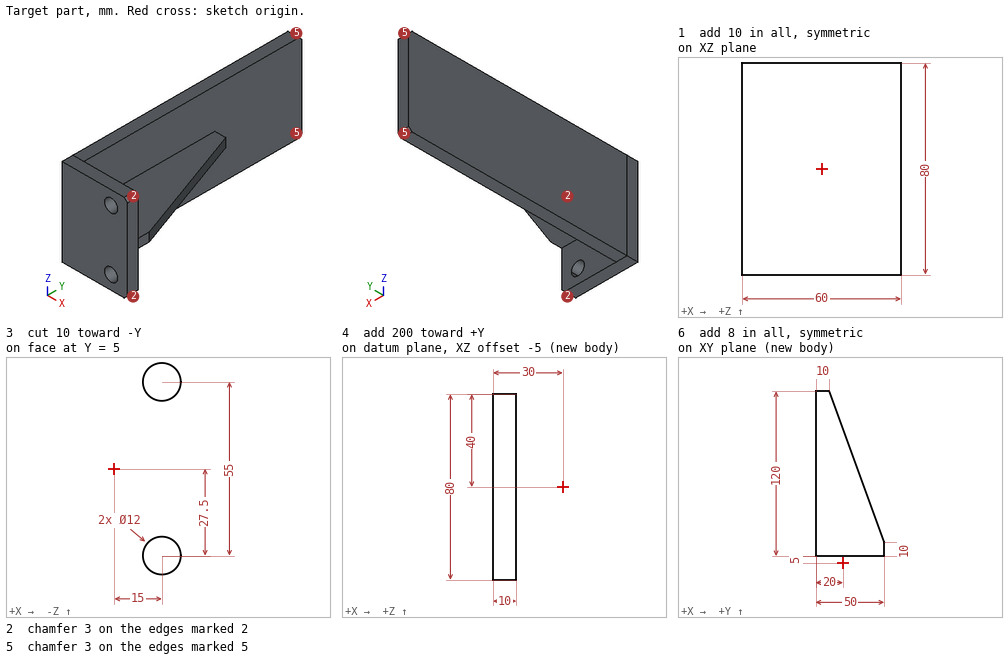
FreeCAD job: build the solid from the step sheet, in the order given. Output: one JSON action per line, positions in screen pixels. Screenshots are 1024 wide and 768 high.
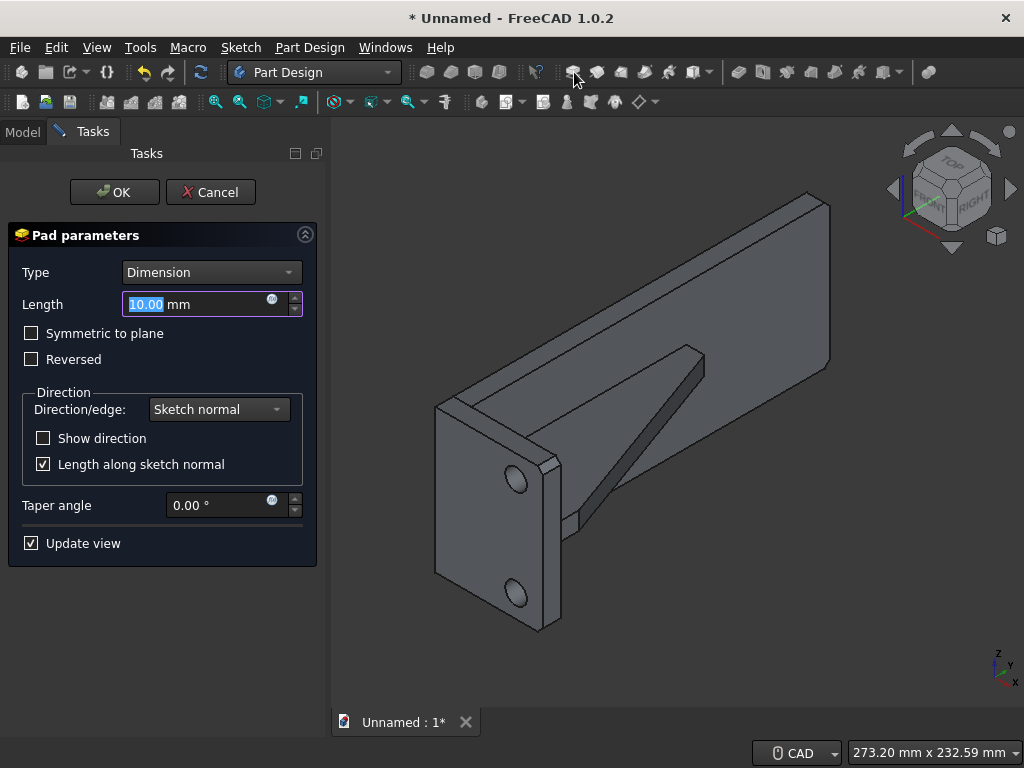
{"action": "type", "text": "8"}
{"action": "key", "text": "Tab"}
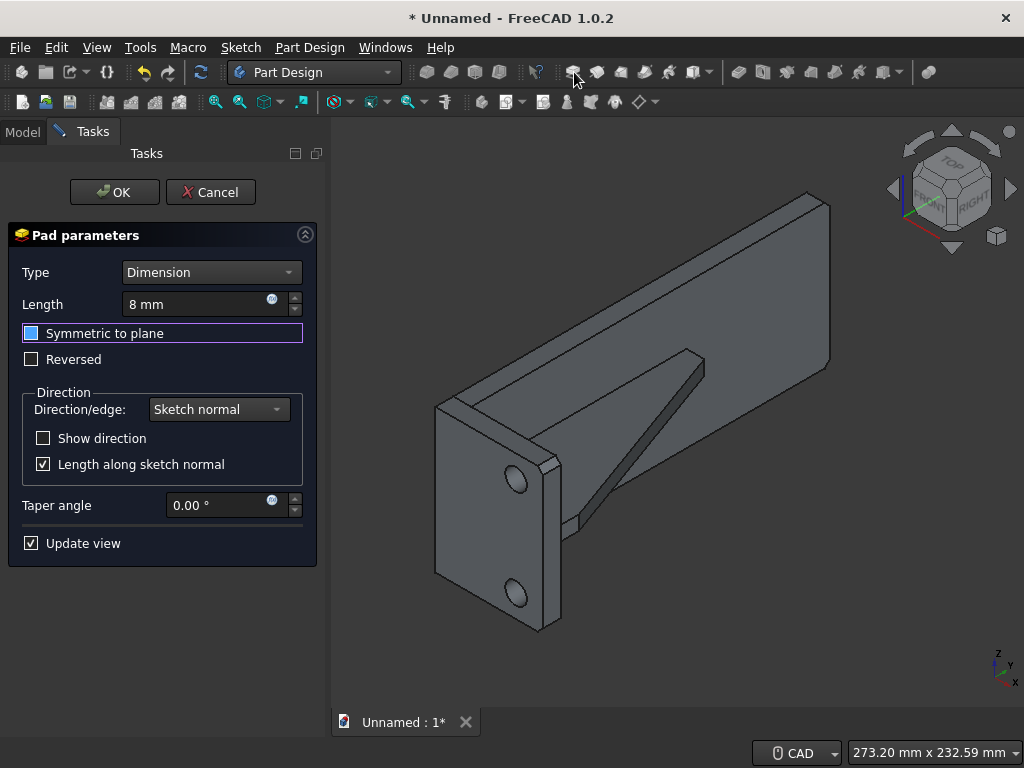
{"action": "left_click", "coordinate": [30, 333]}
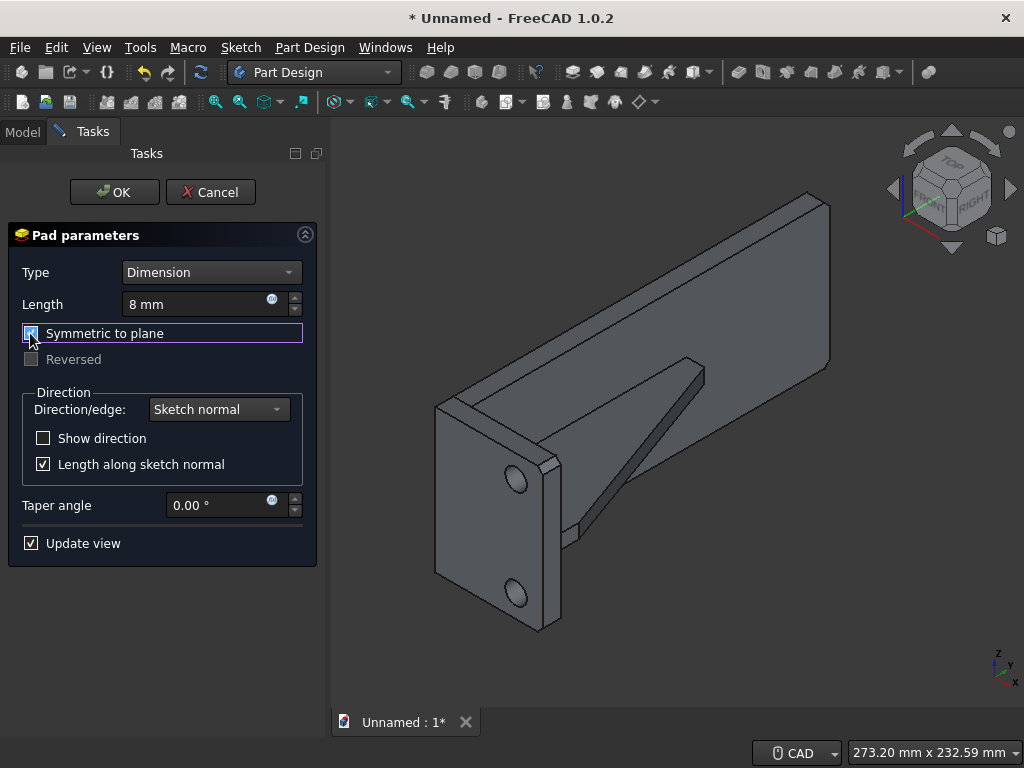
{"action": "left_click", "coordinate": [115, 192]}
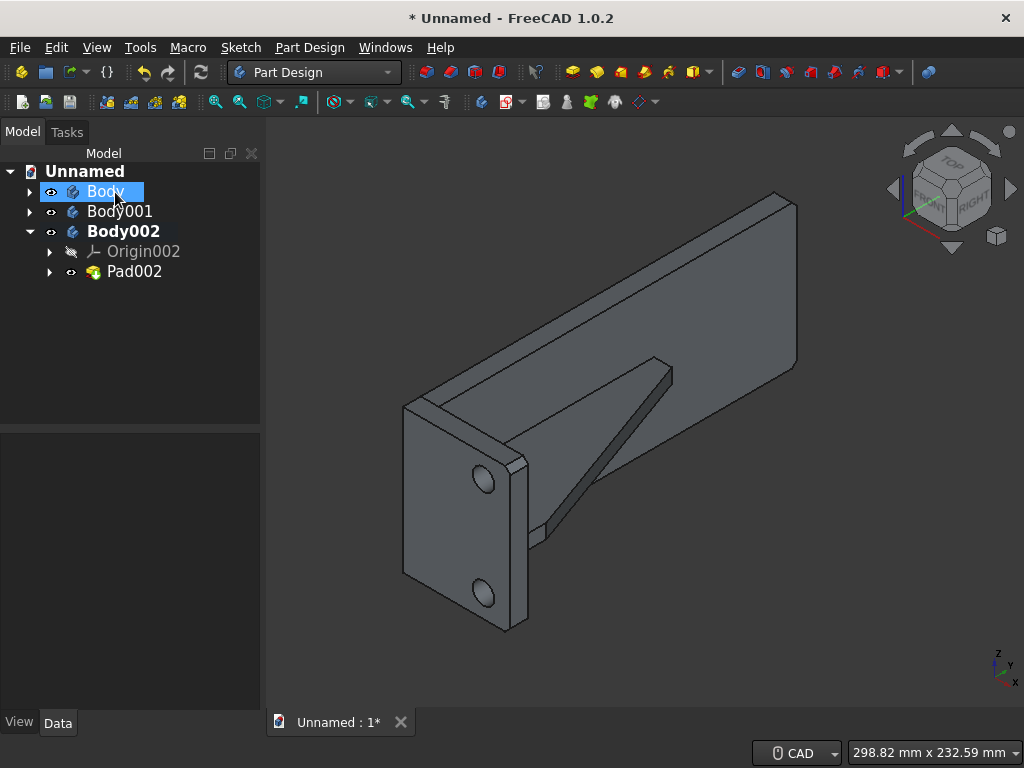
{"action": "left_click", "coordinate": [216, 102]}